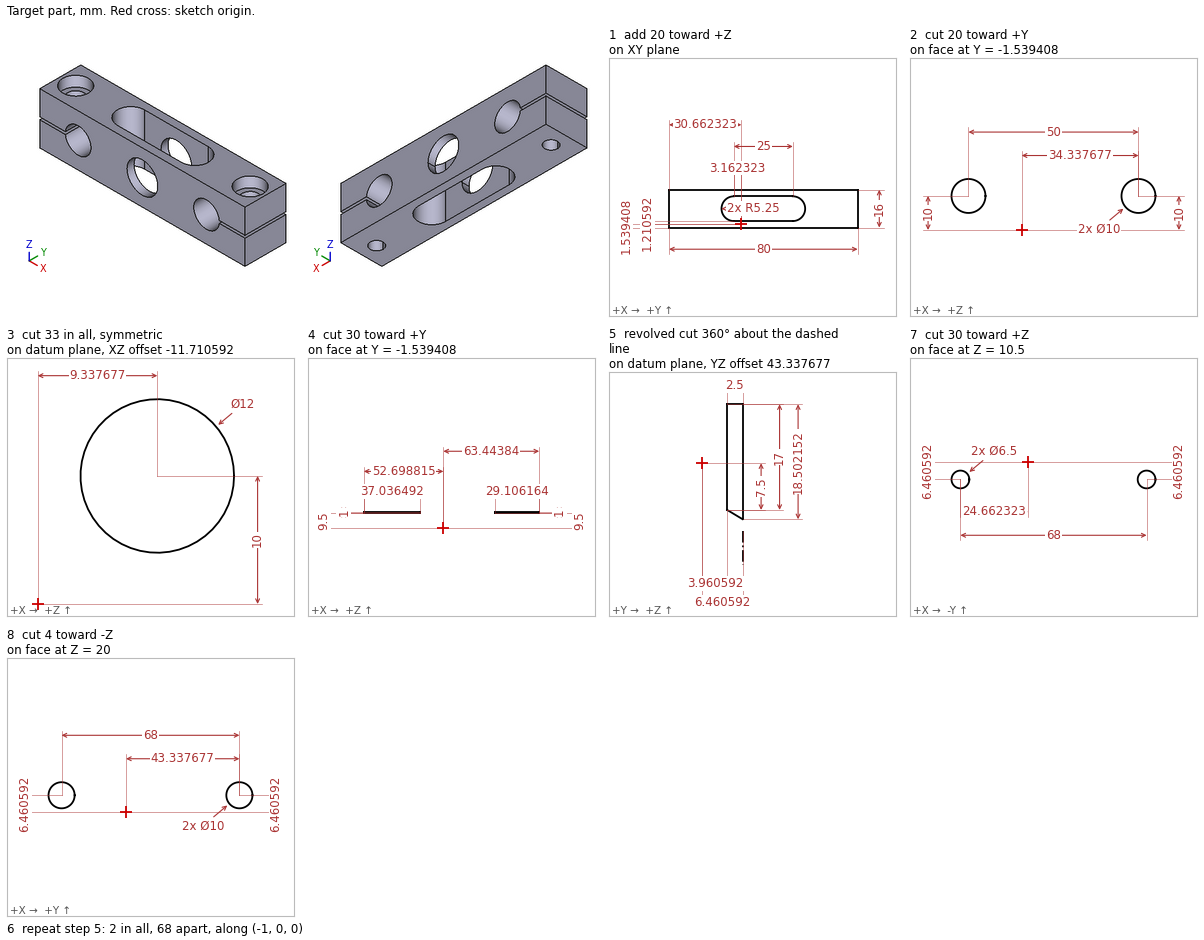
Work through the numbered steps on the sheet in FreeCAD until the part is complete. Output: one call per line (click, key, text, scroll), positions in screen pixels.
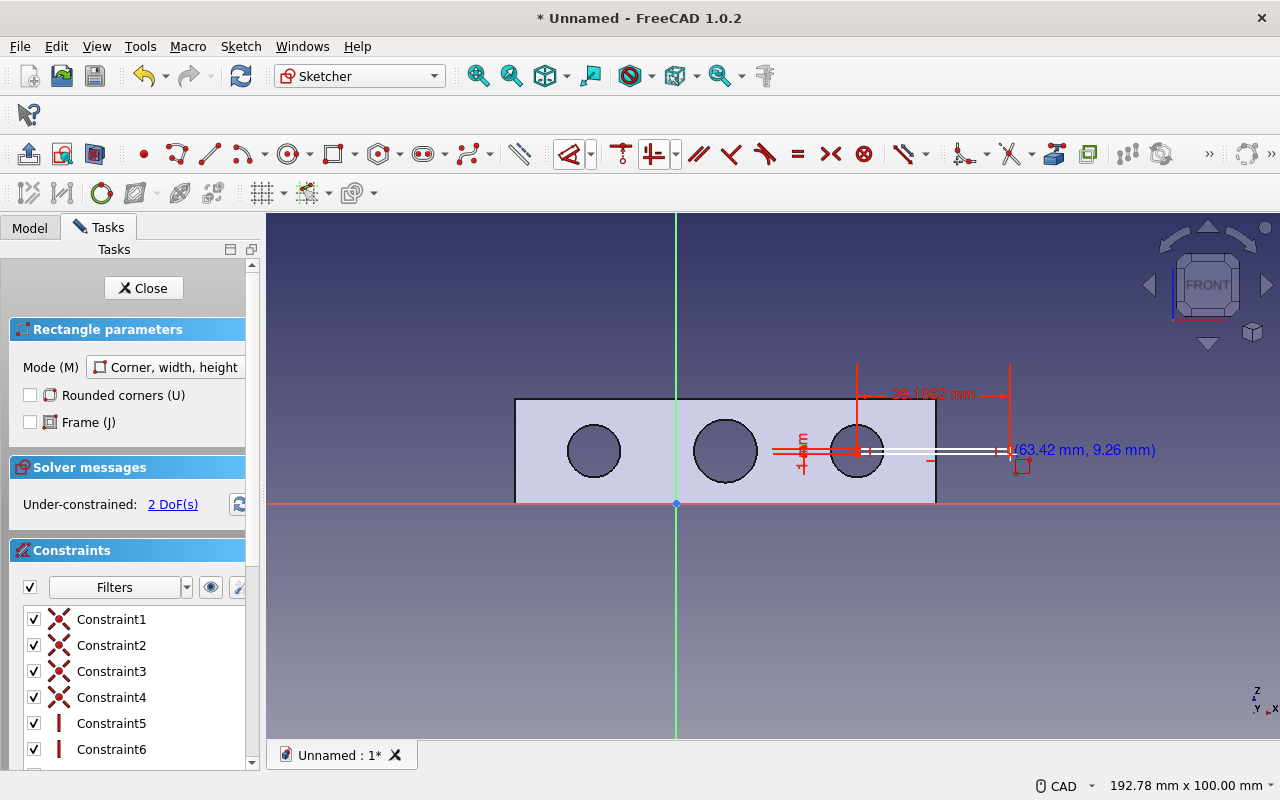
scroll(399, 448, up, 6)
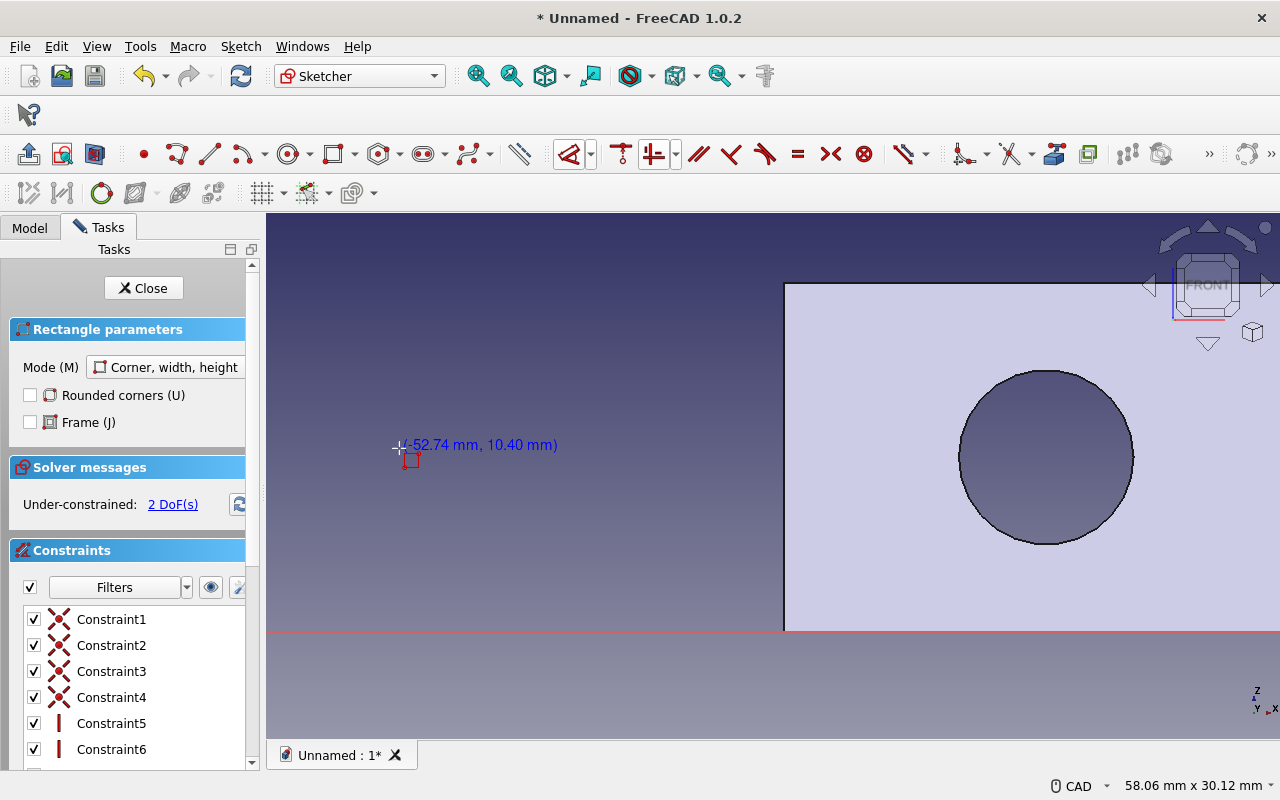
scroll(399, 448, down, 6)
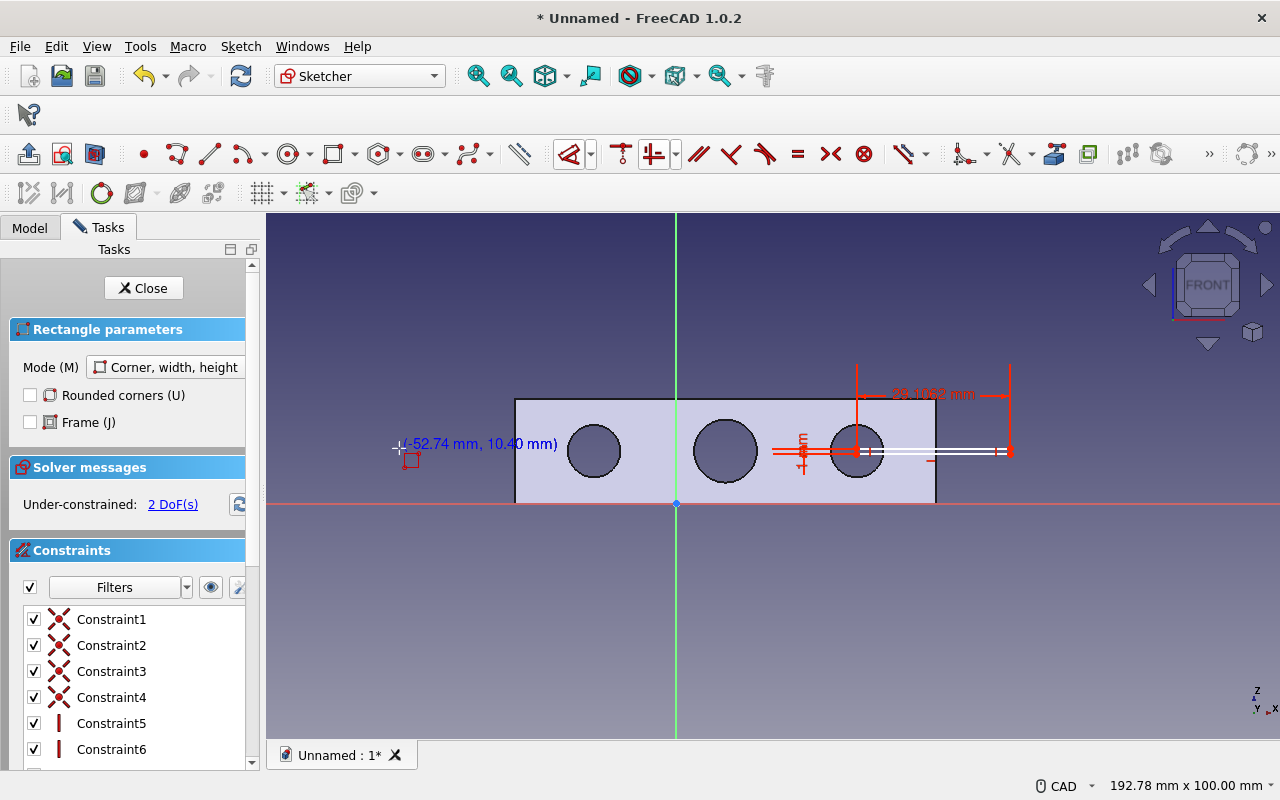
click(399, 448)
move(594, 454)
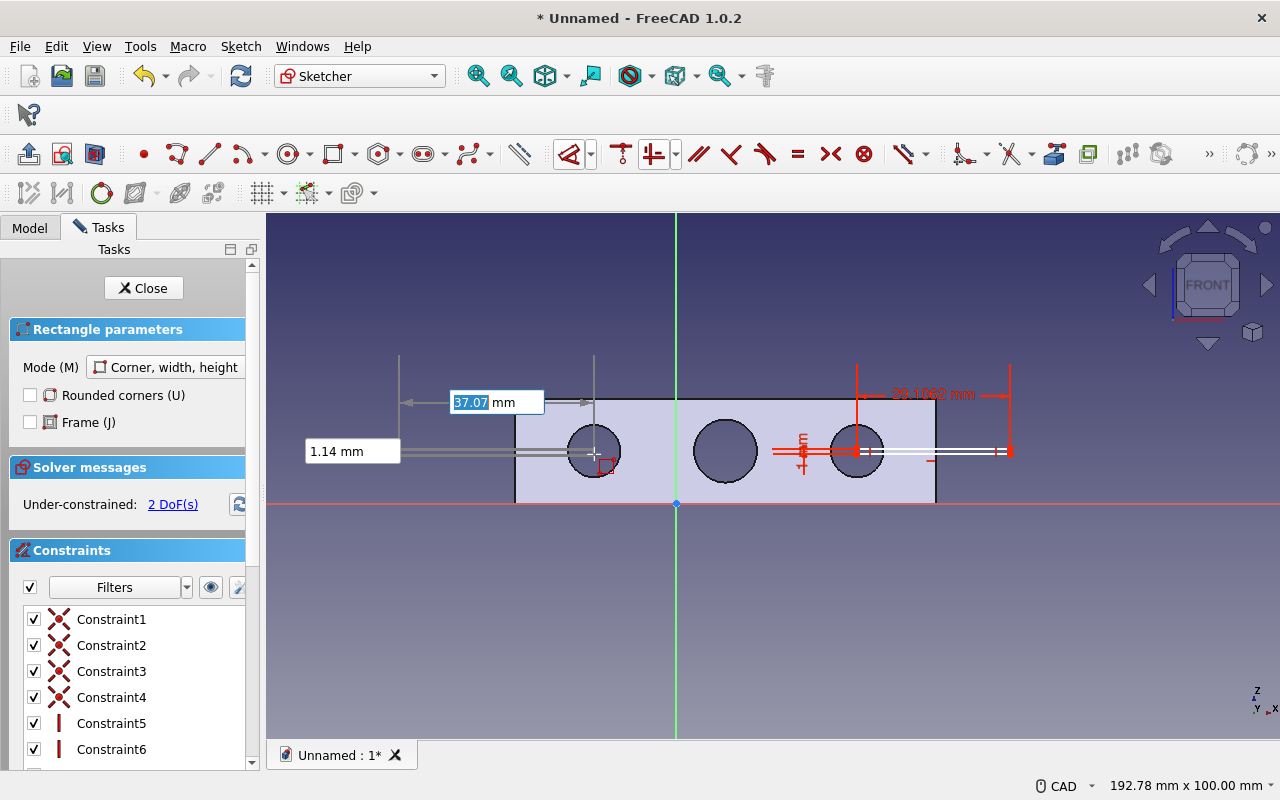
text(37.036492)
key(Tab)
text(1)
key(Return)
key(Escape)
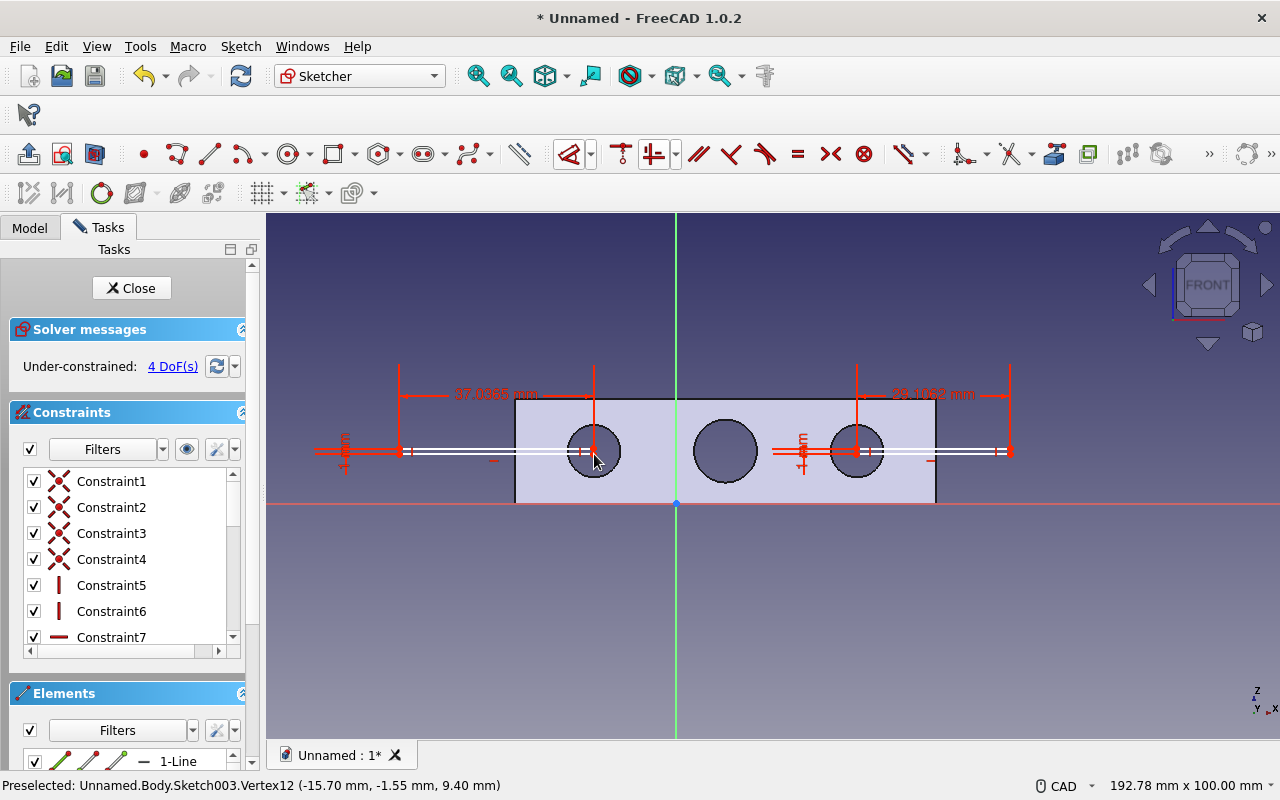
scroll(857, 454, up, 5)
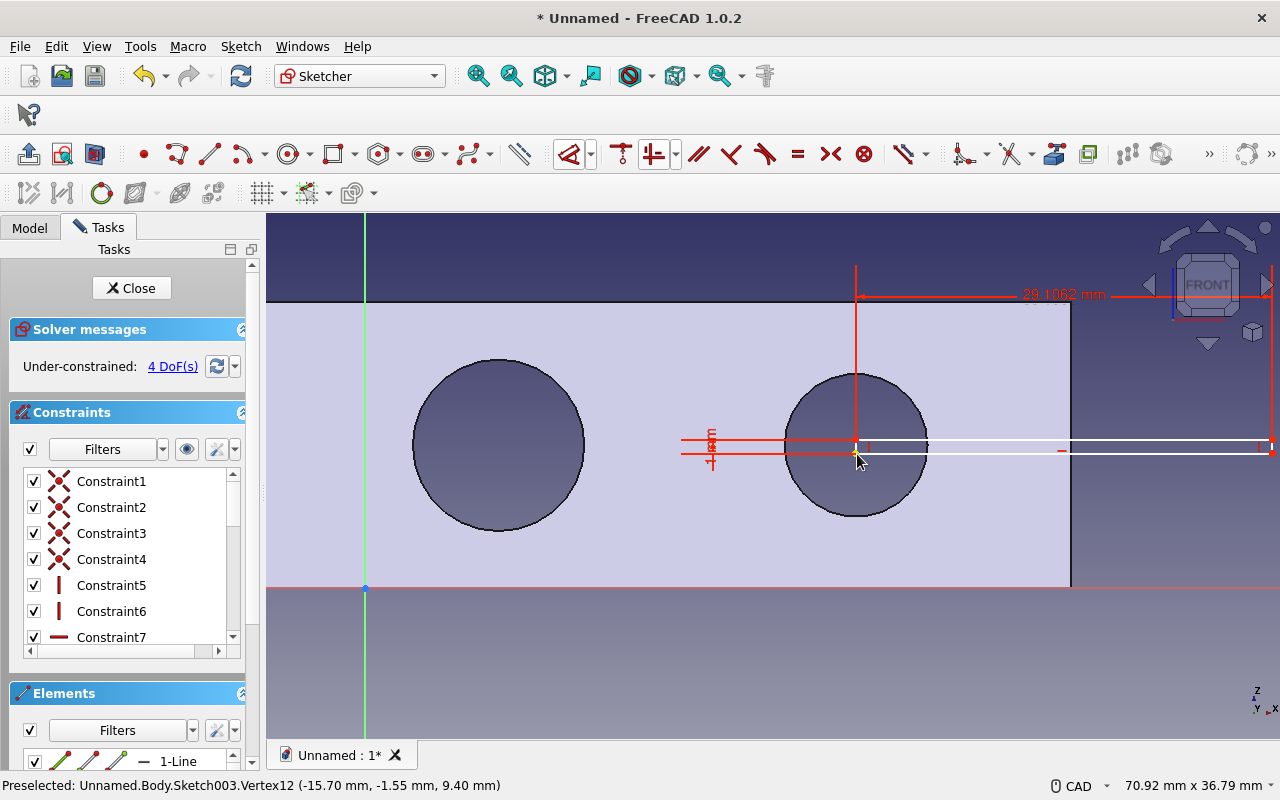
click(856, 454)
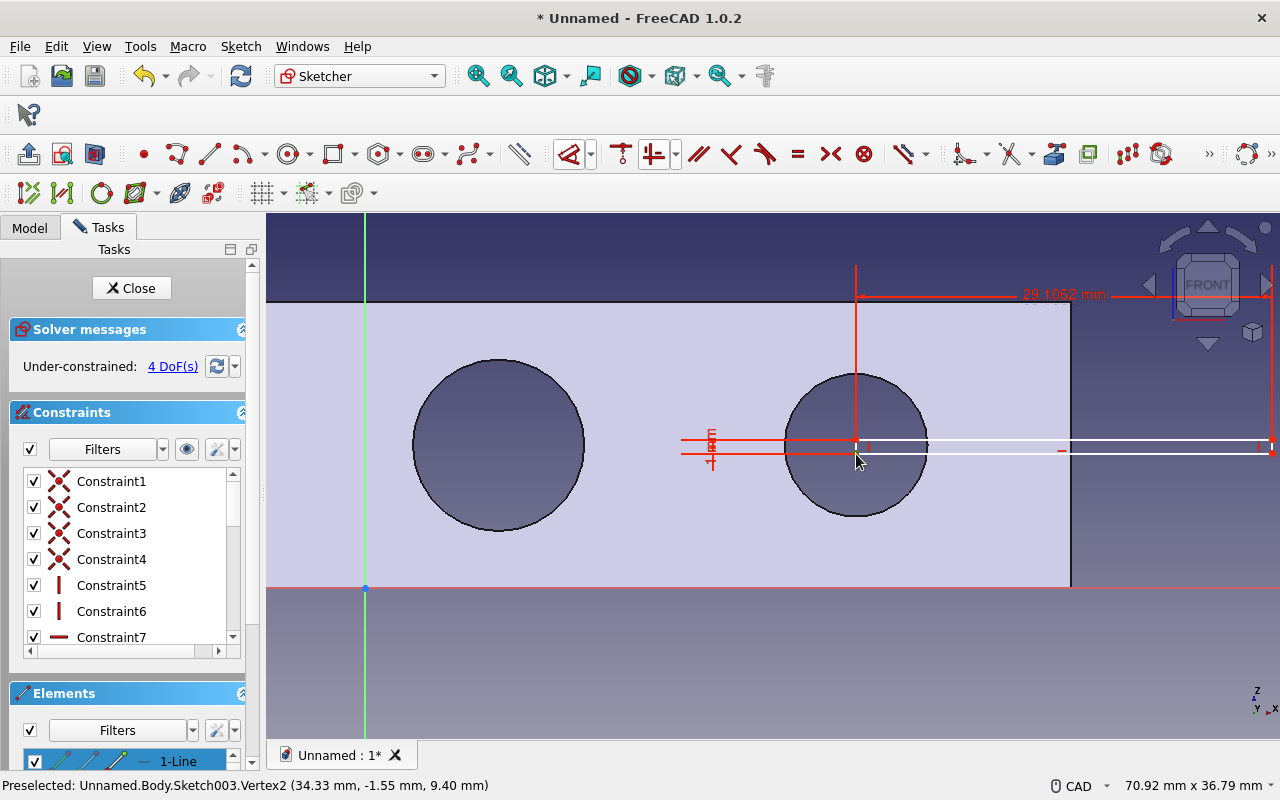
key(i)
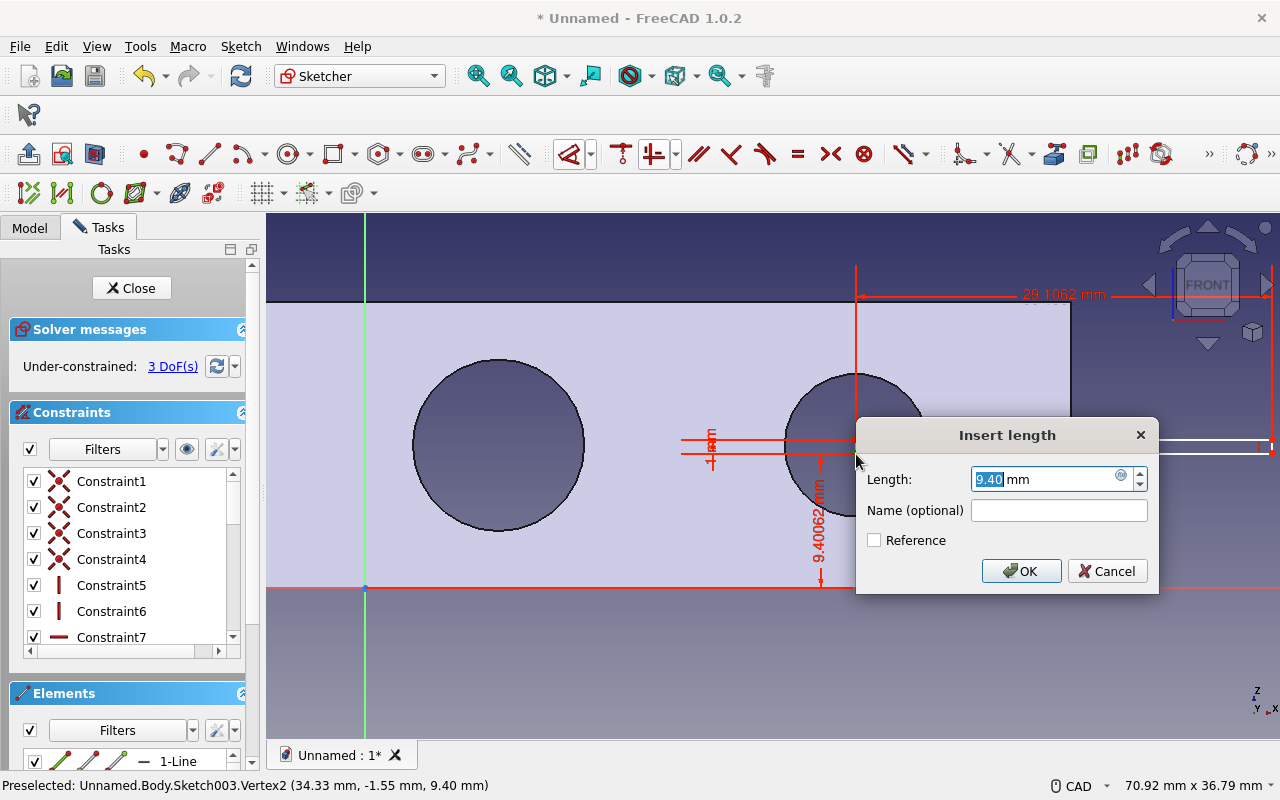
text(9.5)
key(Return)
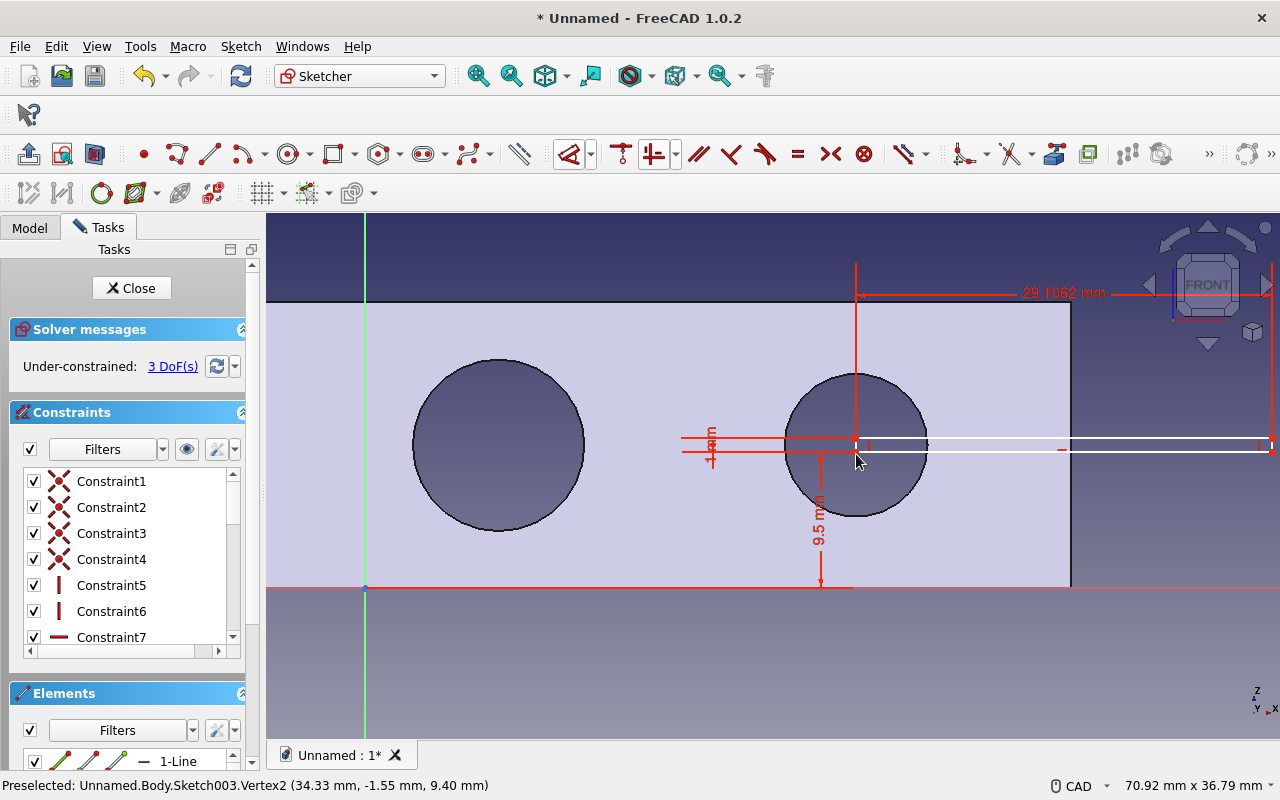
scroll(857, 454, down, 5)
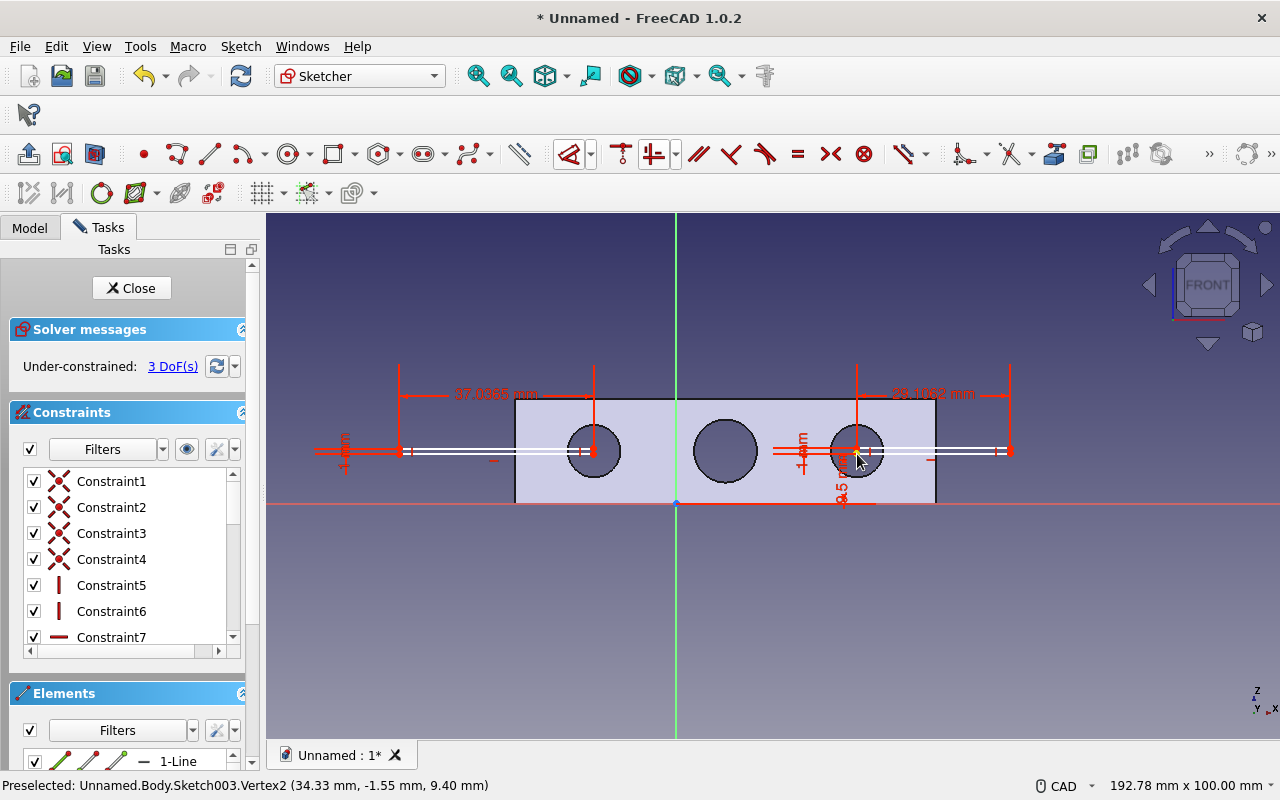
scroll(399, 454, up, 5)